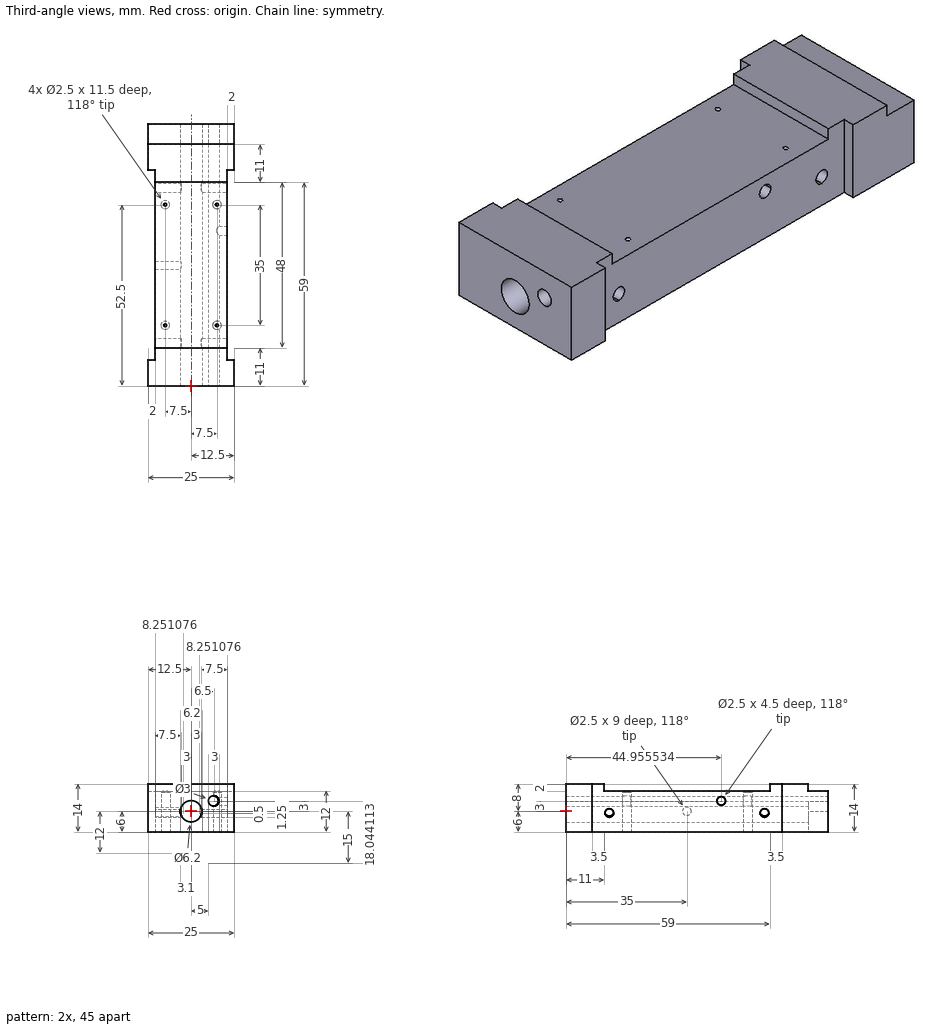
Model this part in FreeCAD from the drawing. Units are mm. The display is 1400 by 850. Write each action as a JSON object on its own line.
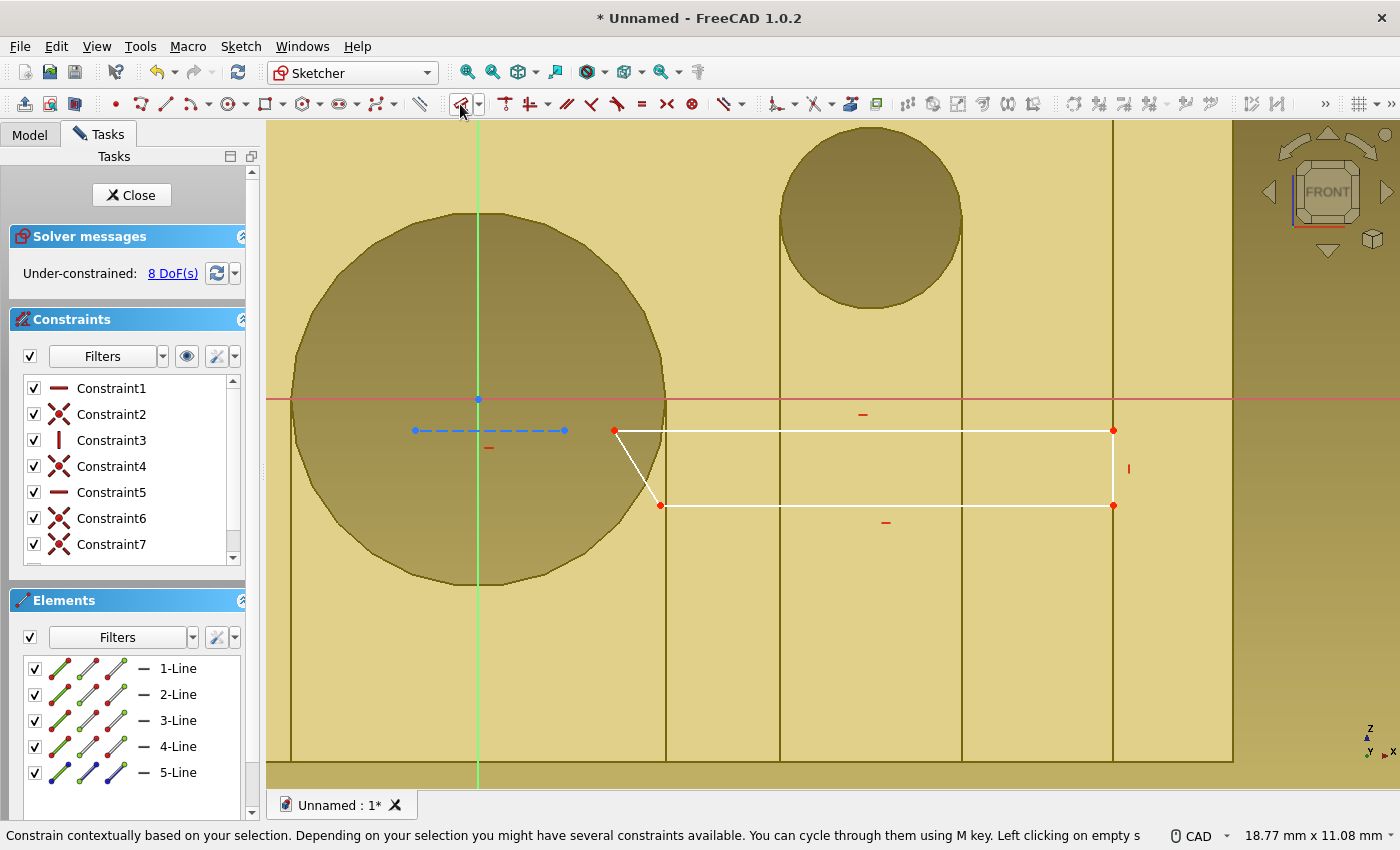
{"action": "left_click", "coordinate": [660, 506]}
{"action": "left_click", "coordinate": [569, 540]}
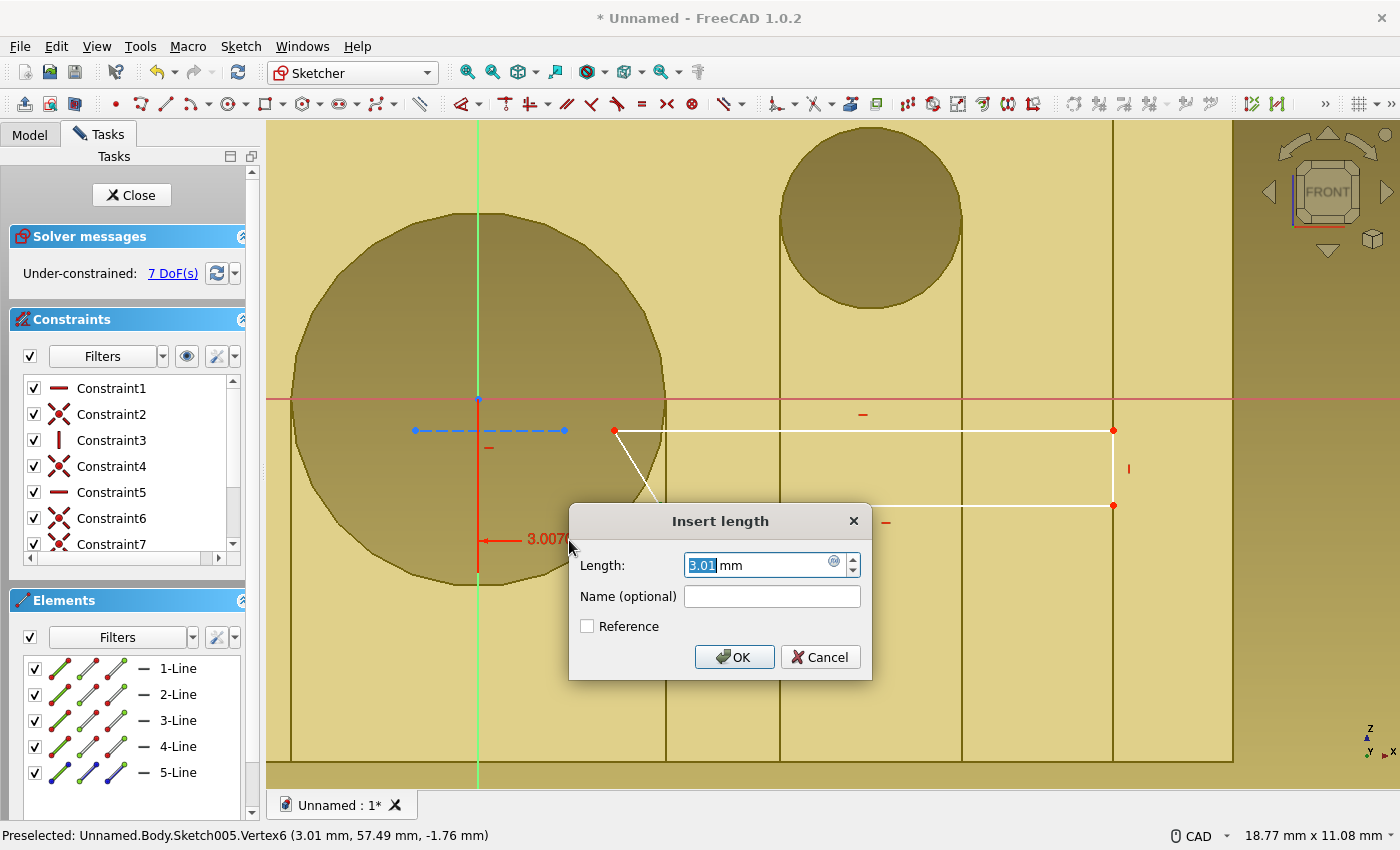
{"action": "type", "text": "3"}
{"action": "key", "text": "Return"}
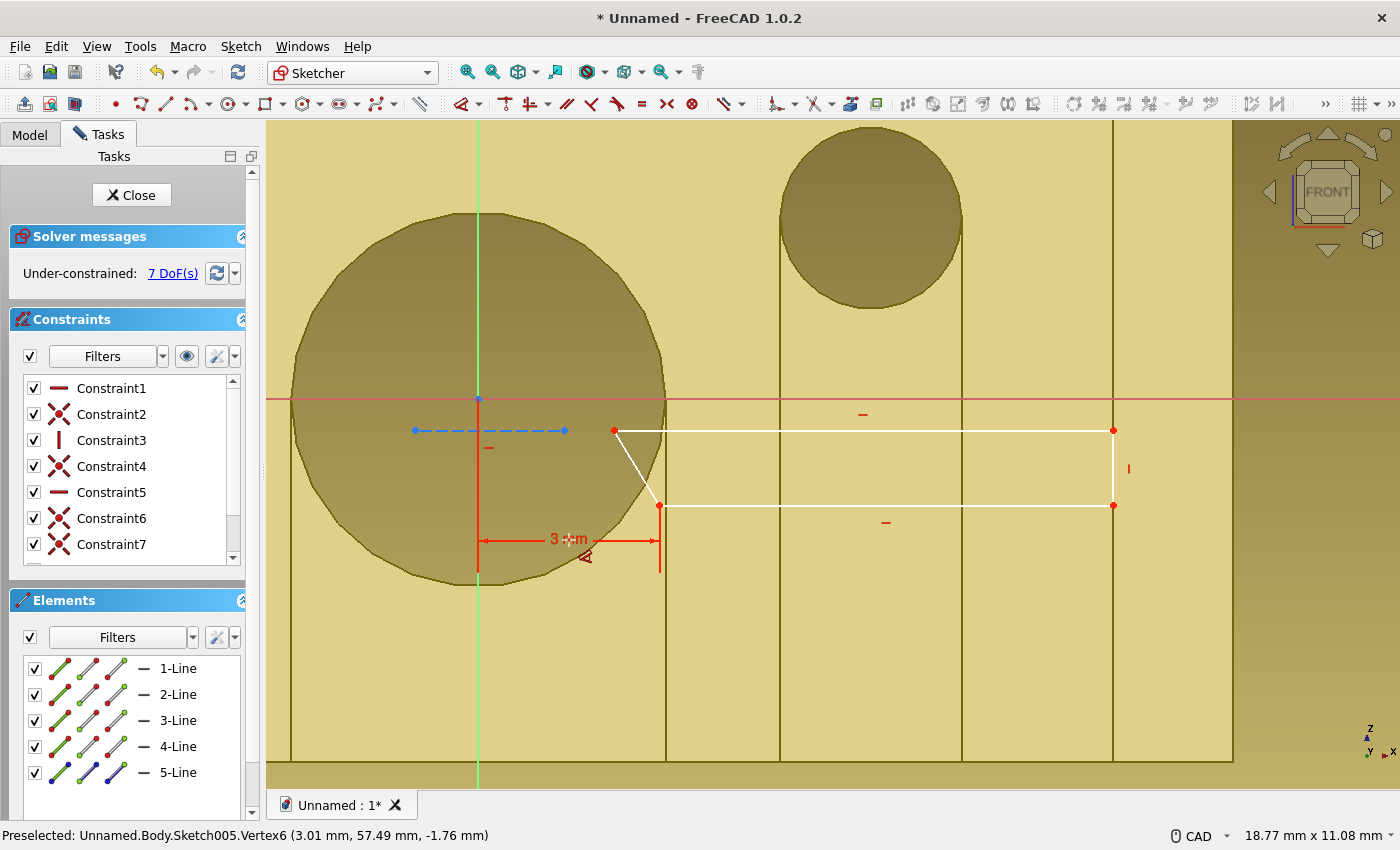
{"action": "left_click", "coordinate": [977, 506]}
{"action": "left_click", "coordinate": [886, 540]}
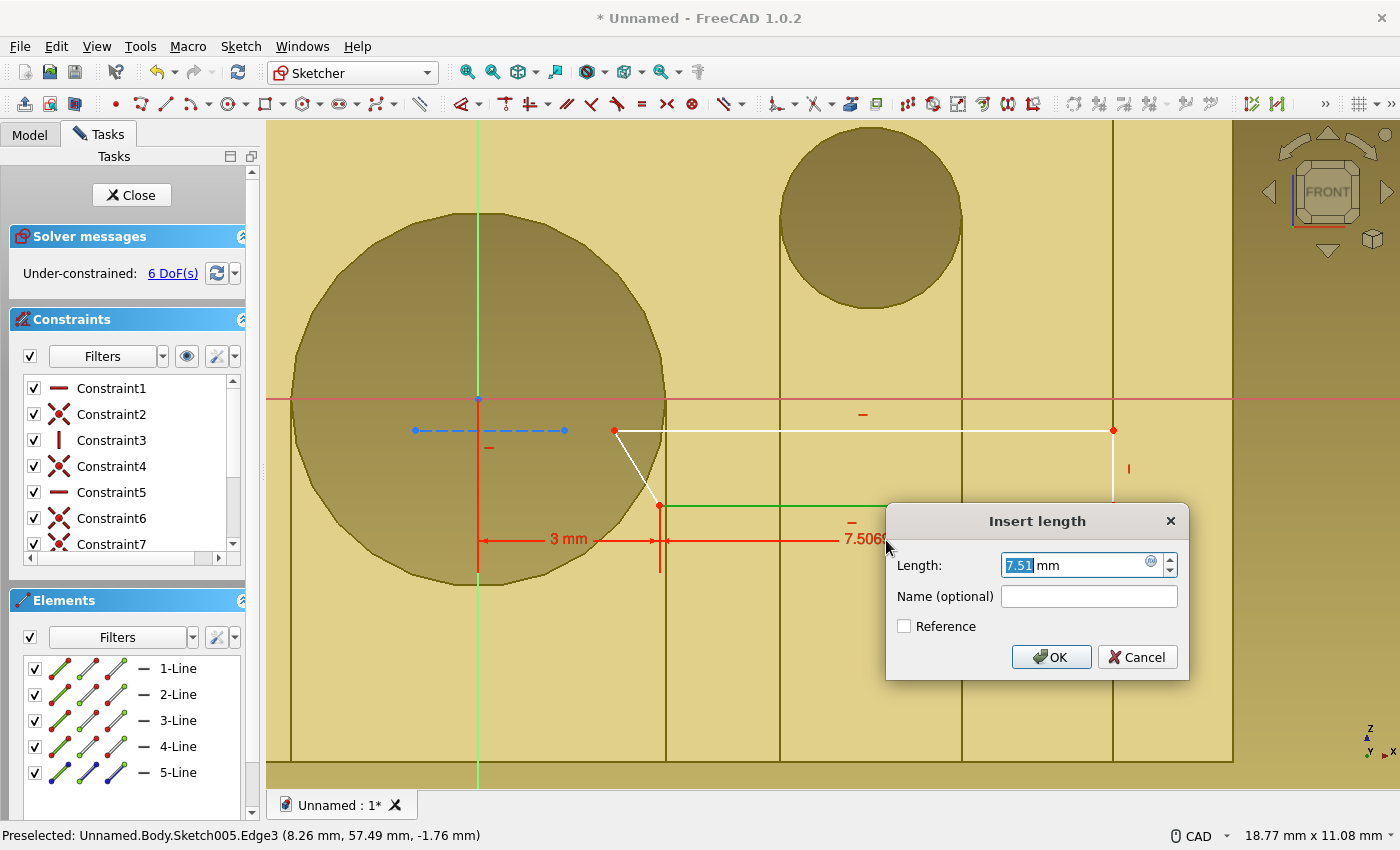
{"action": "type", "text": "7.5"}
{"action": "key", "text": "Return"}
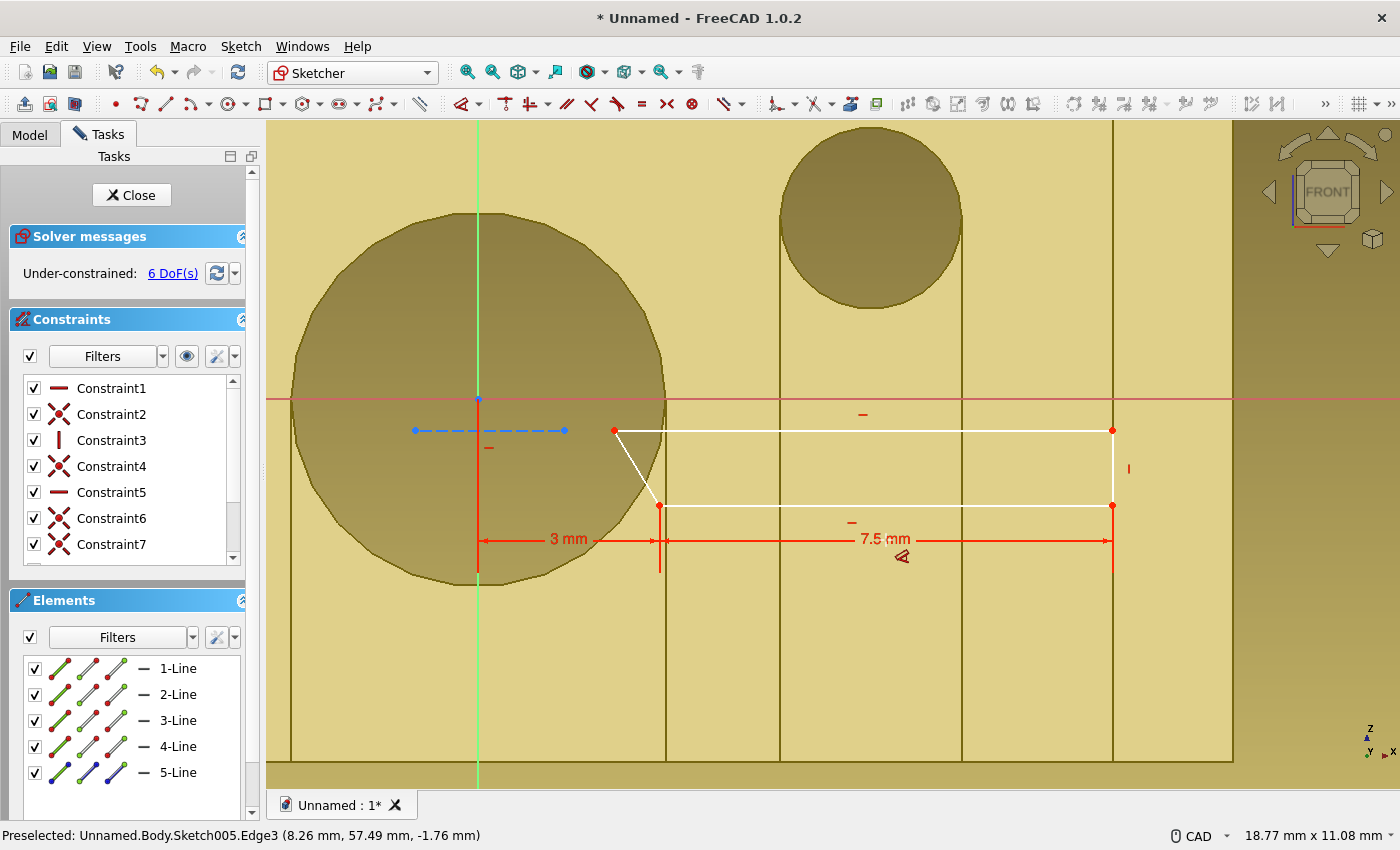
{"action": "left_click", "coordinate": [1113, 454]}
{"action": "left_click", "coordinate": [1147, 469]}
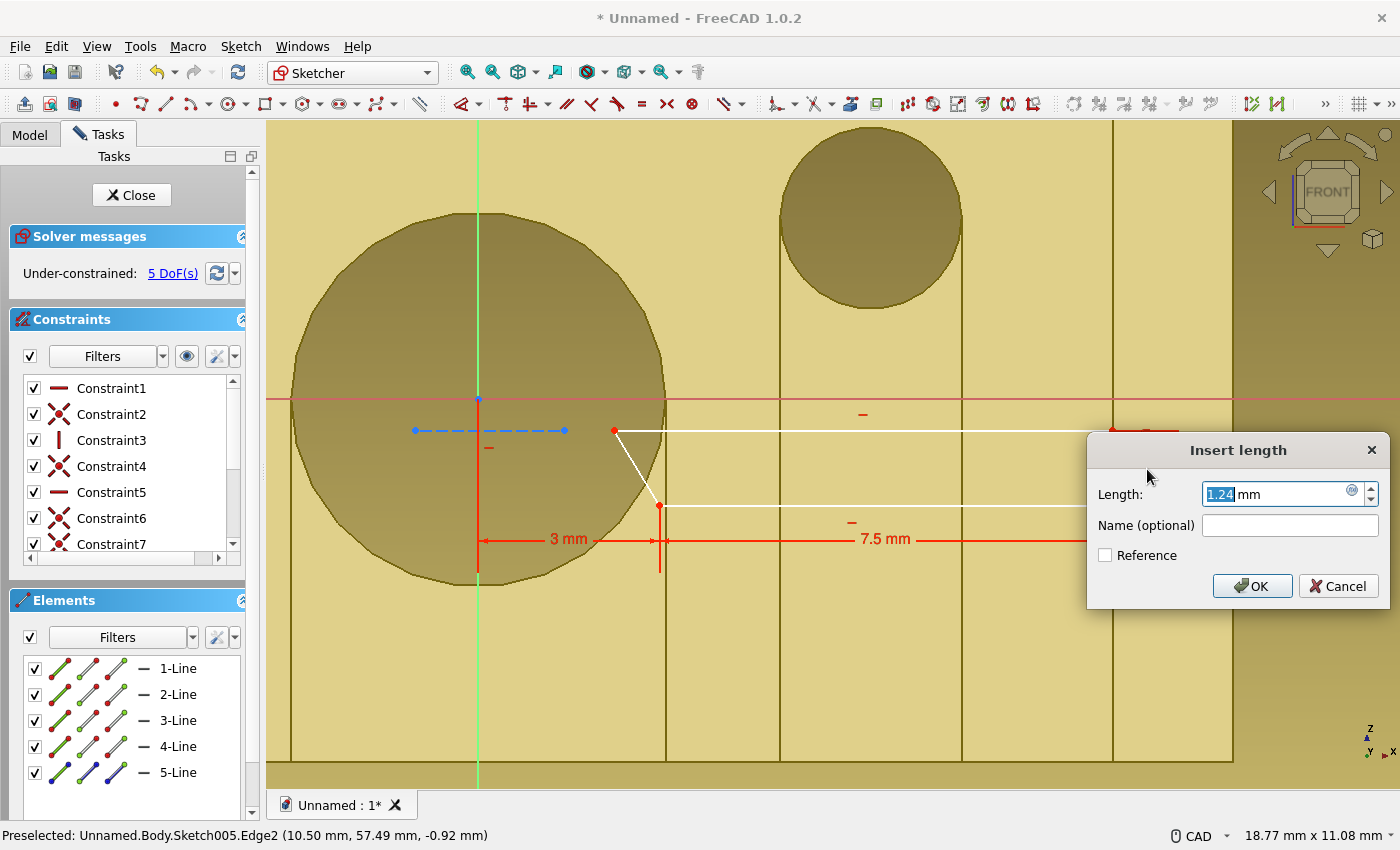
{"action": "type", "text": "1.25"}
{"action": "key", "text": "Return"}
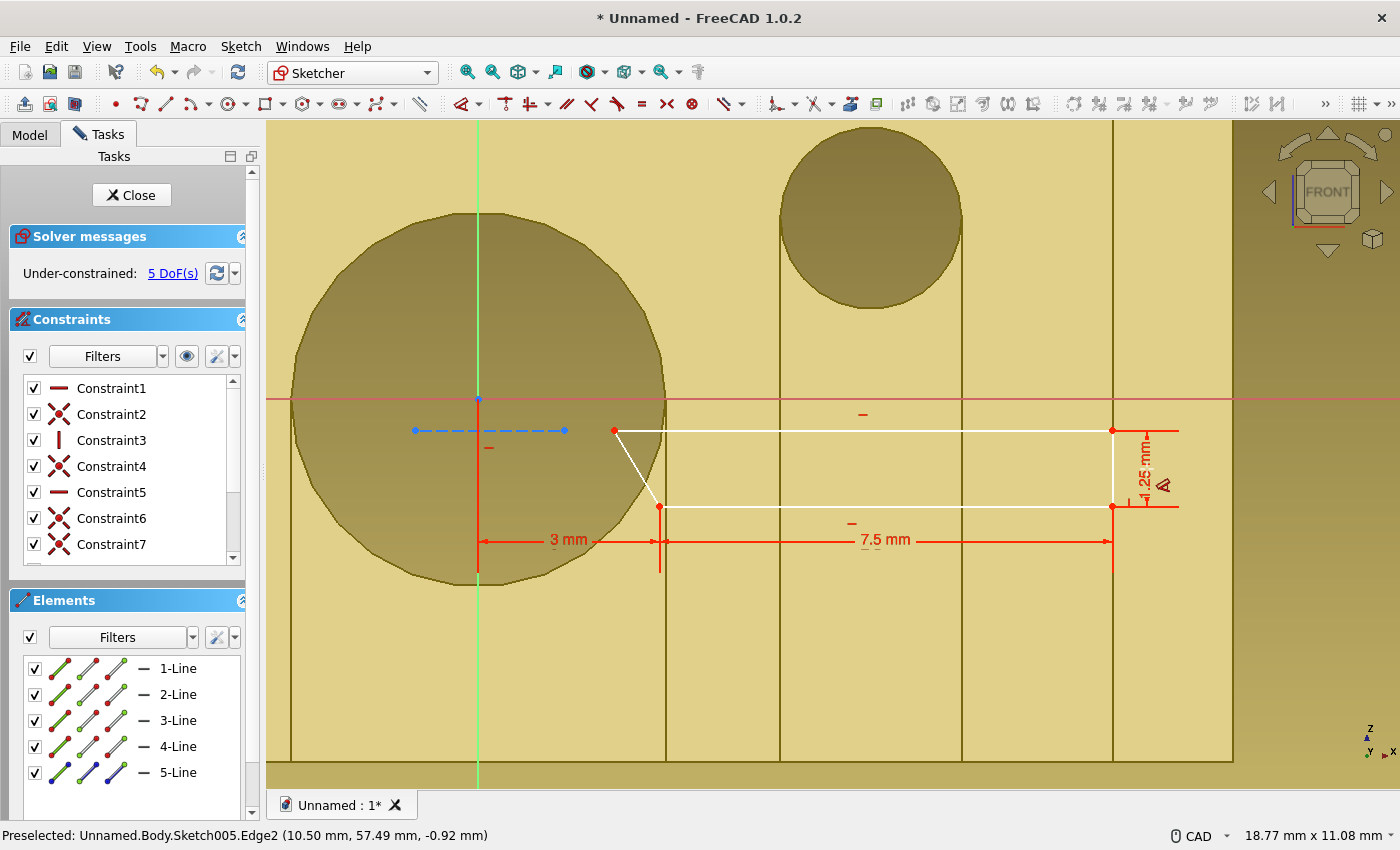
{"action": "scroll", "coordinate": [614, 431], "scroll_direction": "up", "scroll_amount": 2}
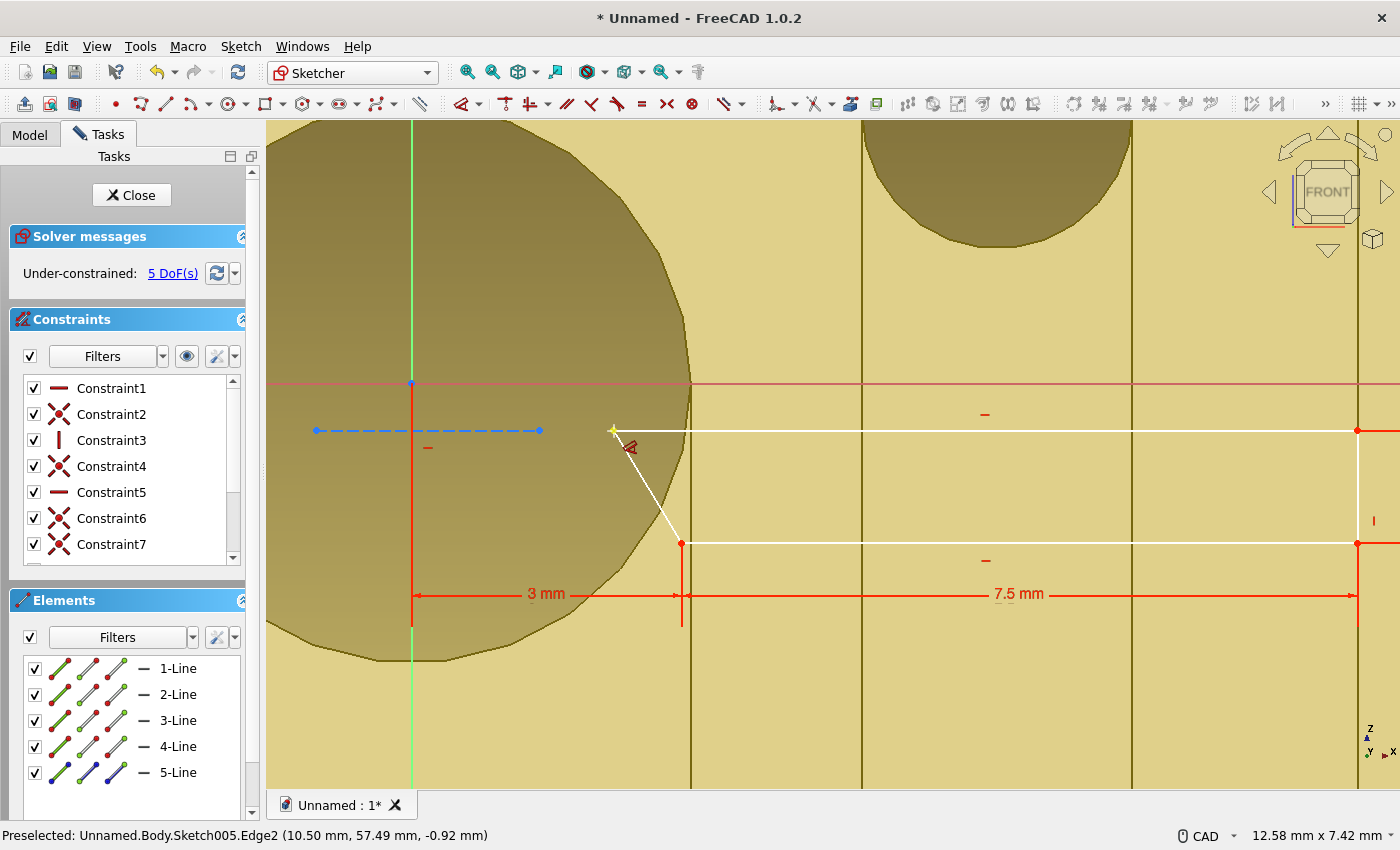
{"action": "left_click", "coordinate": [614, 431]}
{"action": "left_click", "coordinate": [378, 407]}